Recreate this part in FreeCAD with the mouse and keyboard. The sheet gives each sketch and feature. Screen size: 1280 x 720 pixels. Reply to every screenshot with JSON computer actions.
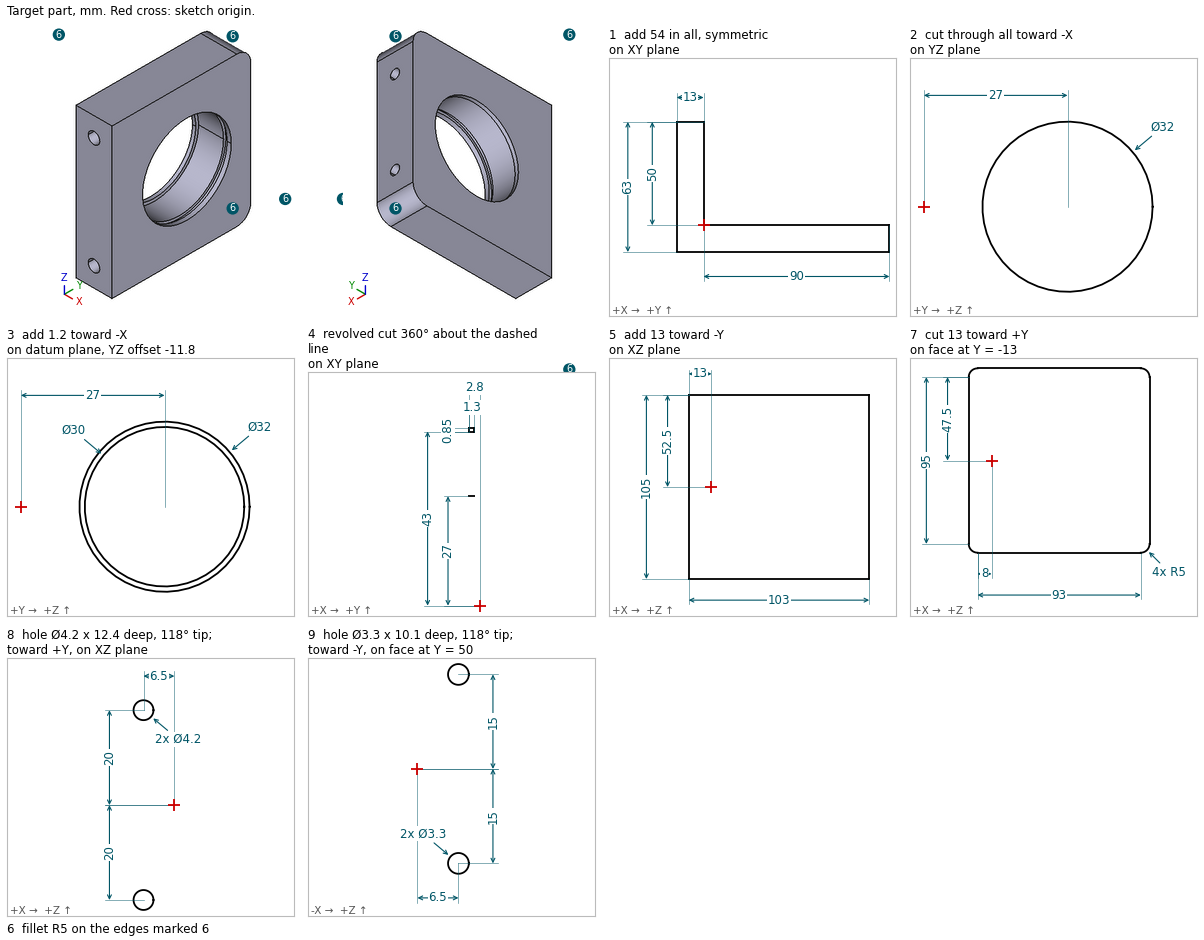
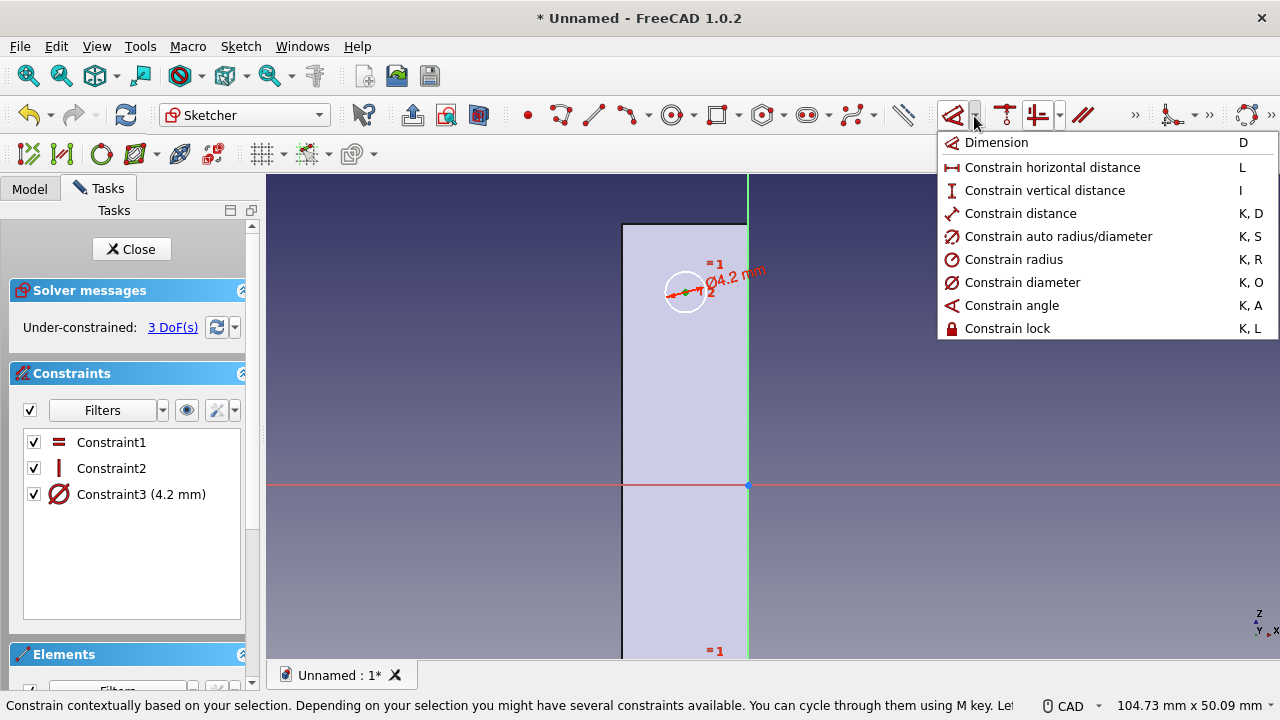
{"action": "left_click", "coordinate": [1108, 190]}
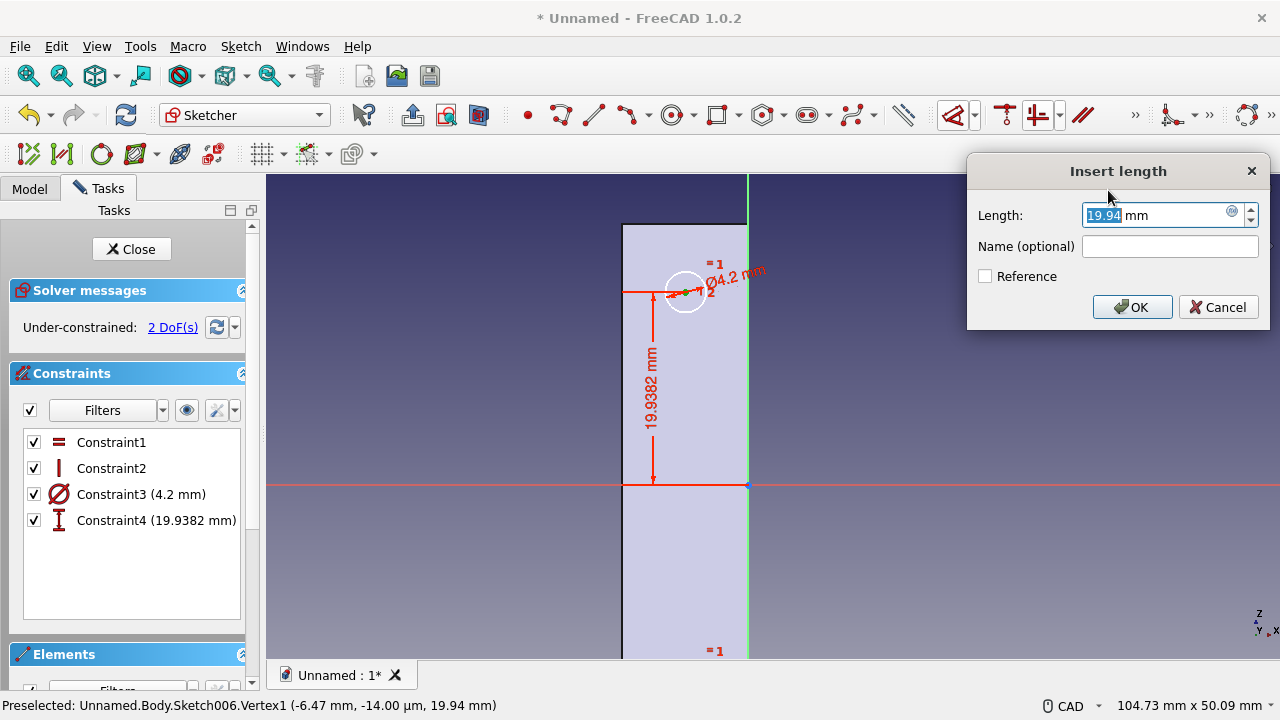
{"action": "type", "text": "20"}
{"action": "key", "text": "Return"}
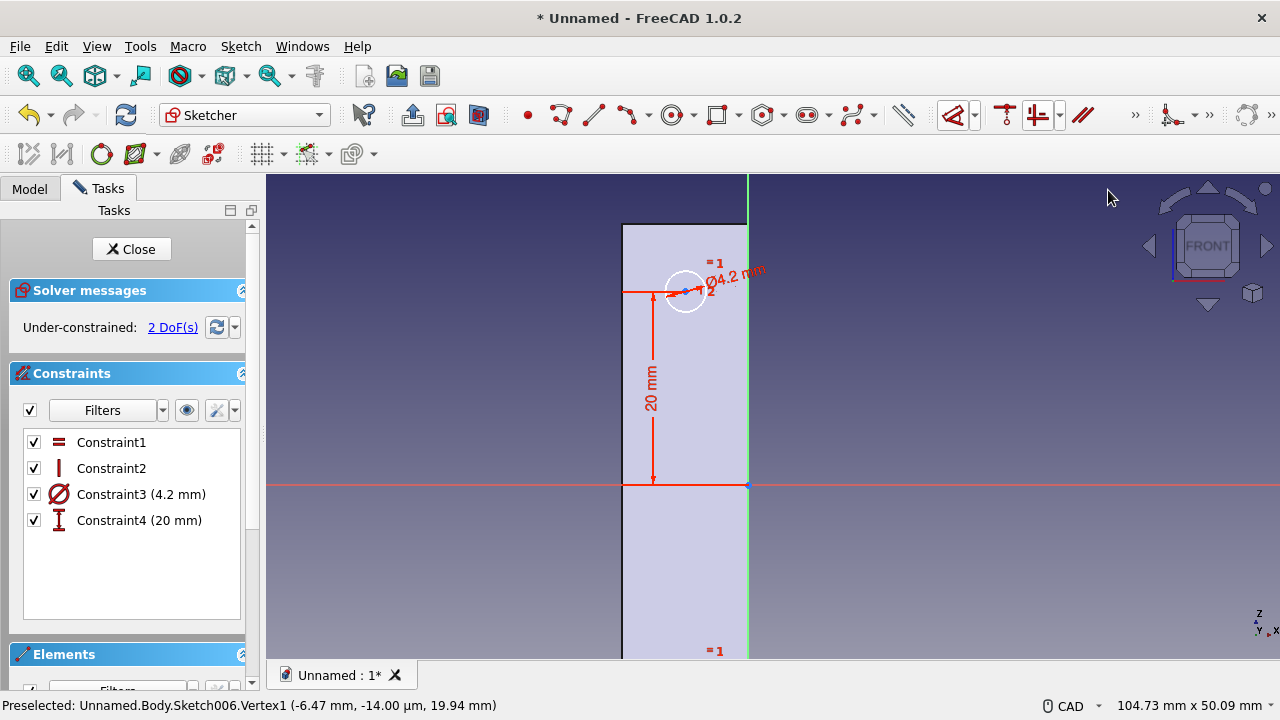
{"action": "scroll", "coordinate": [700, 277], "scroll_direction": "down", "scroll_amount": 2}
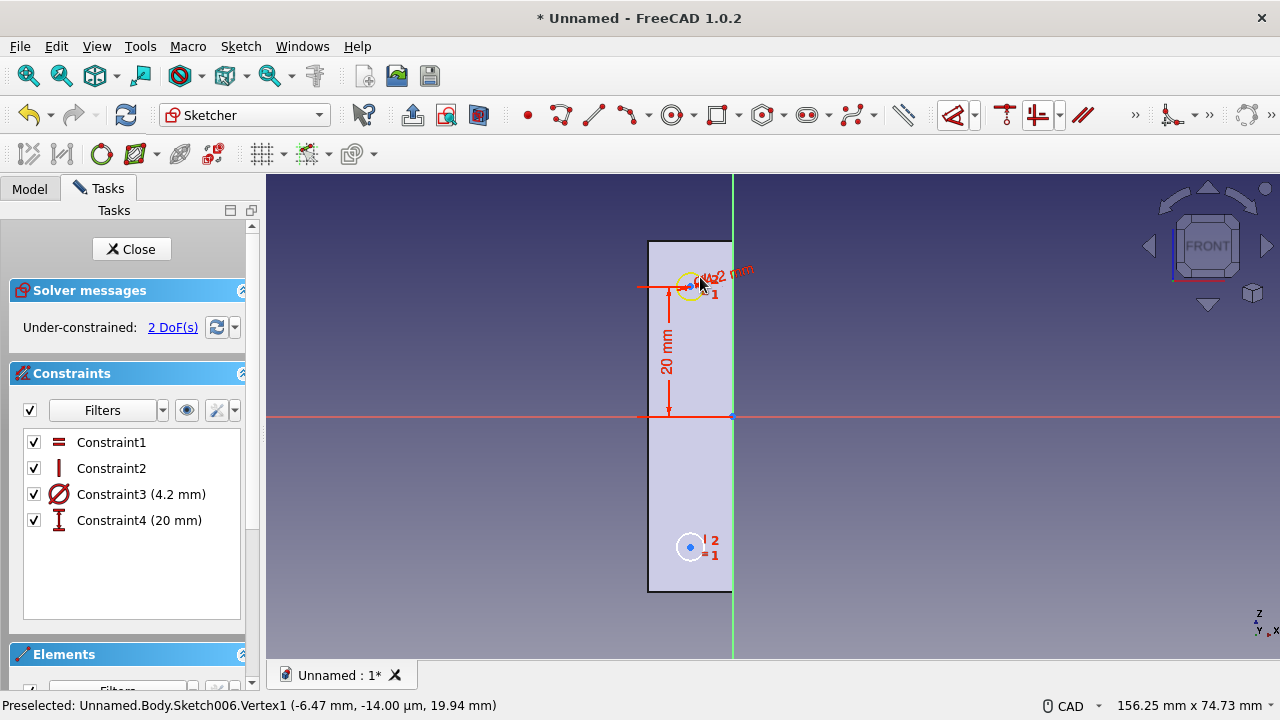
{"action": "left_click", "coordinate": [691, 547]}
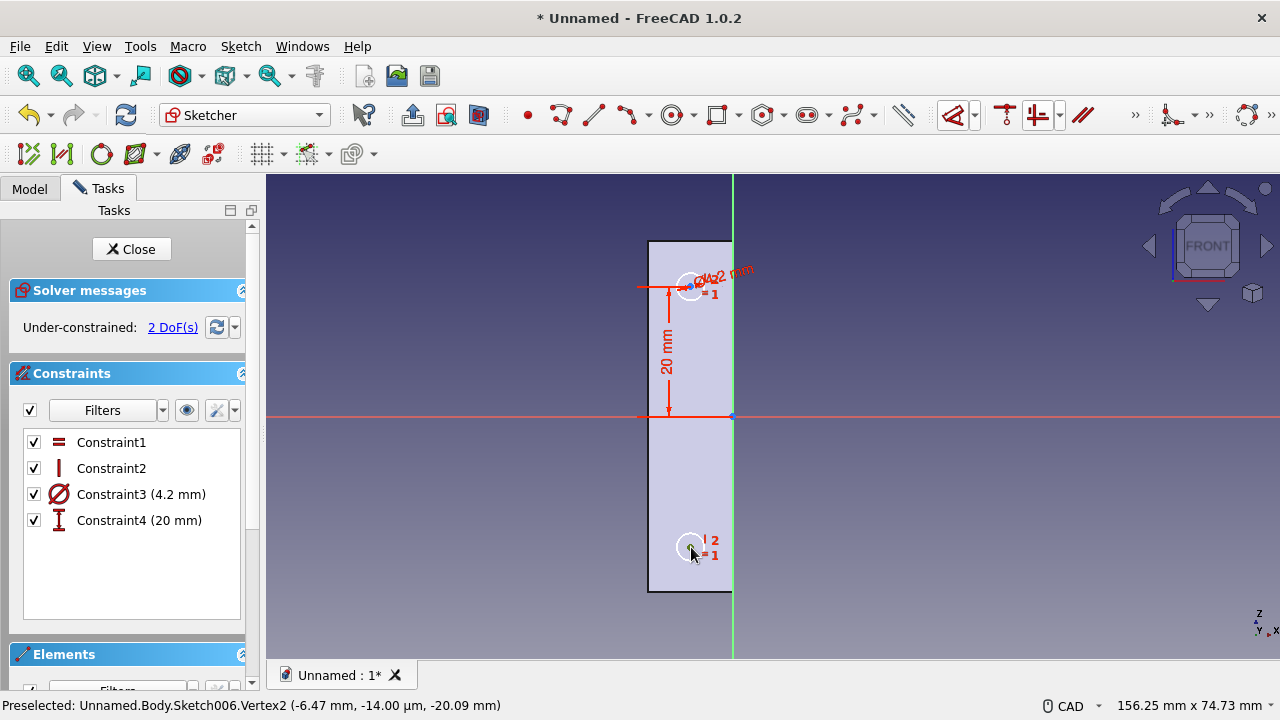
{"action": "left_click", "coordinate": [974, 116]}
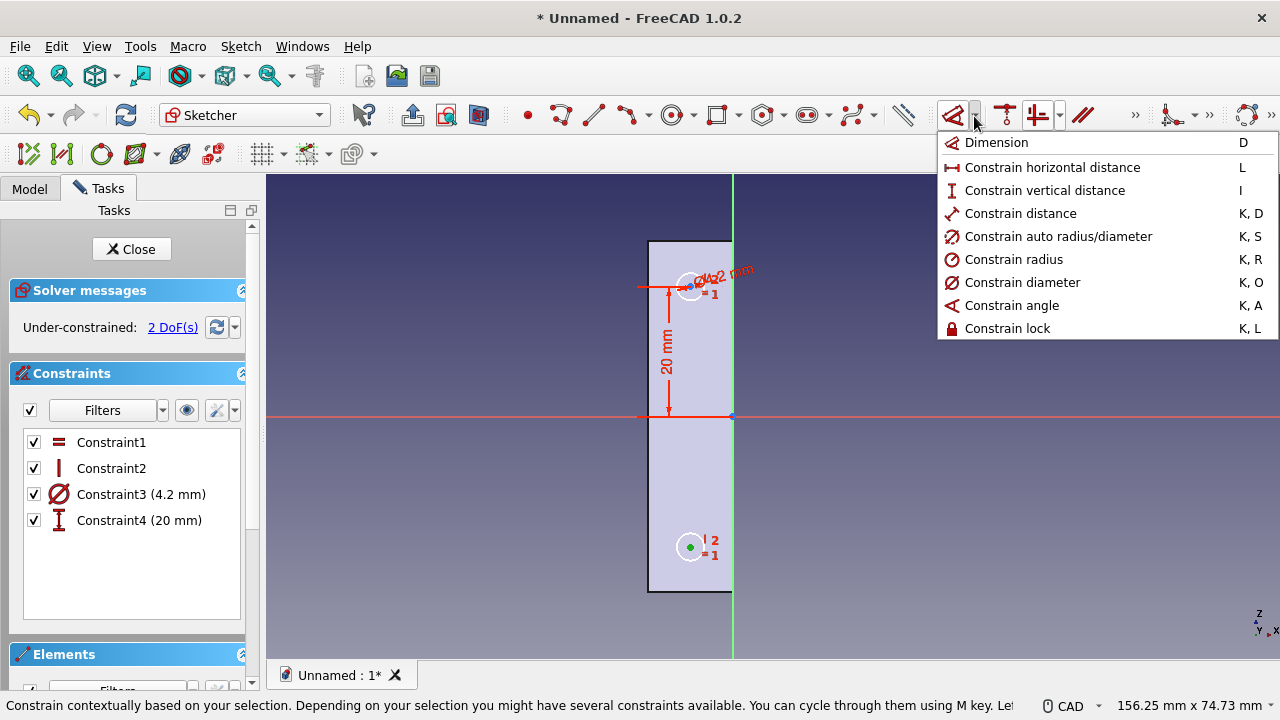
{"action": "left_click", "coordinate": [1108, 190]}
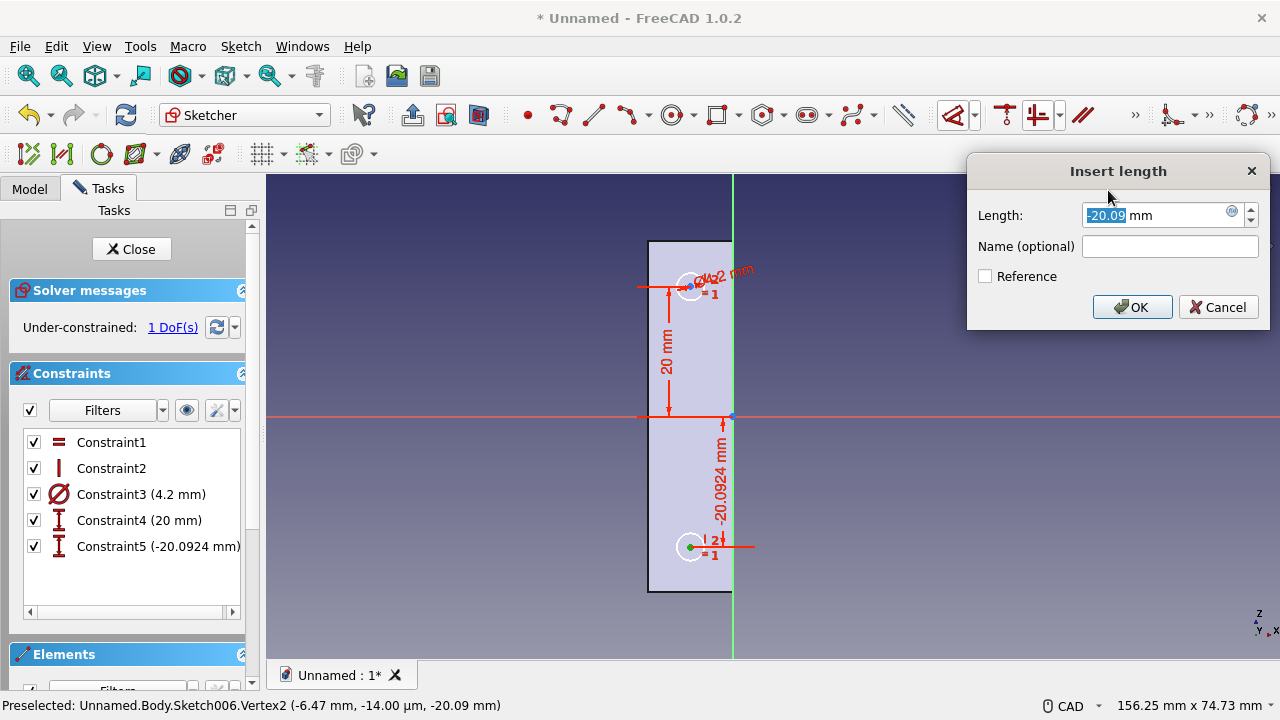
{"action": "type", "text": "-20"}
{"action": "key", "text": "Return"}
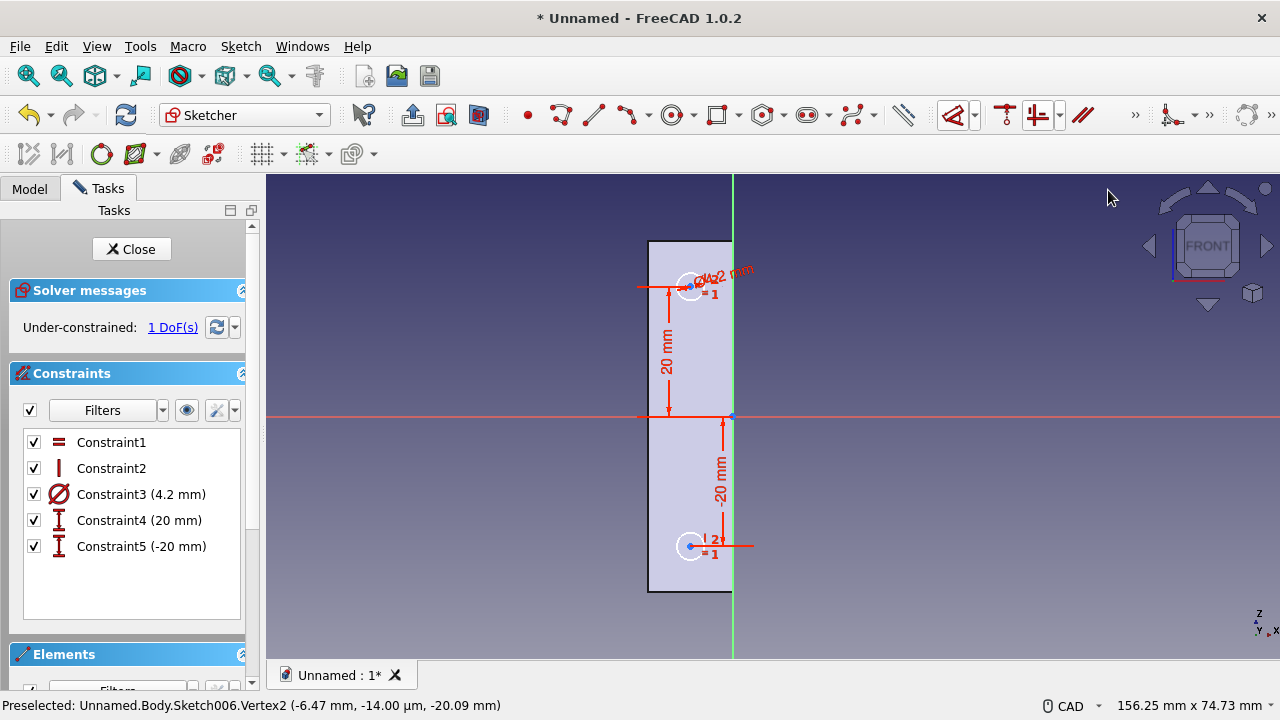
{"action": "left_click", "coordinate": [691, 287]}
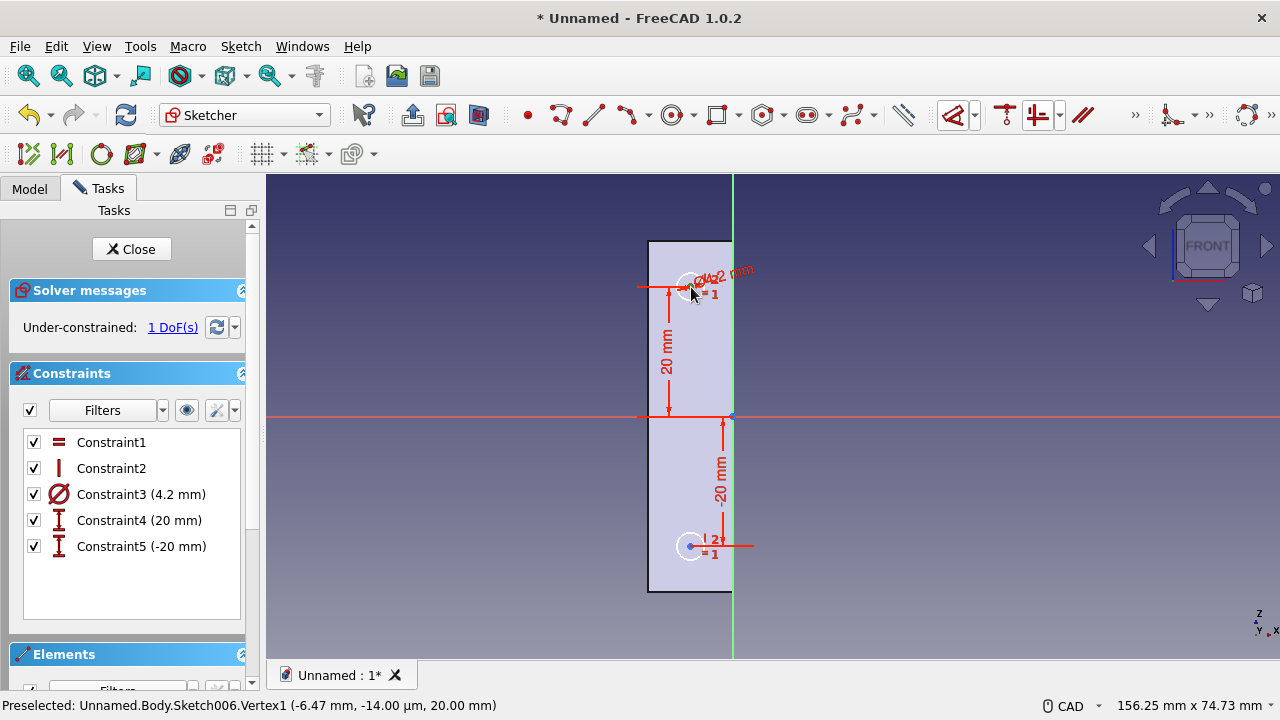
{"action": "left_click", "coordinate": [974, 116]}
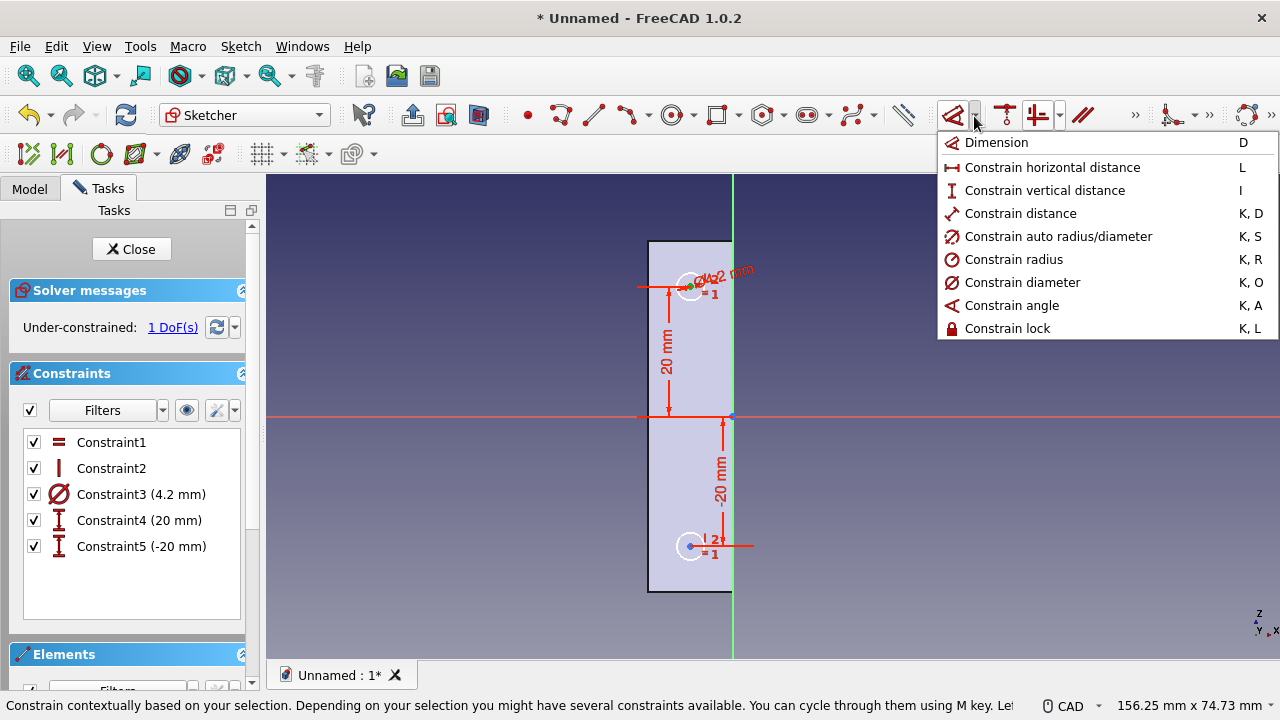
{"action": "left_click", "coordinate": [1108, 168]}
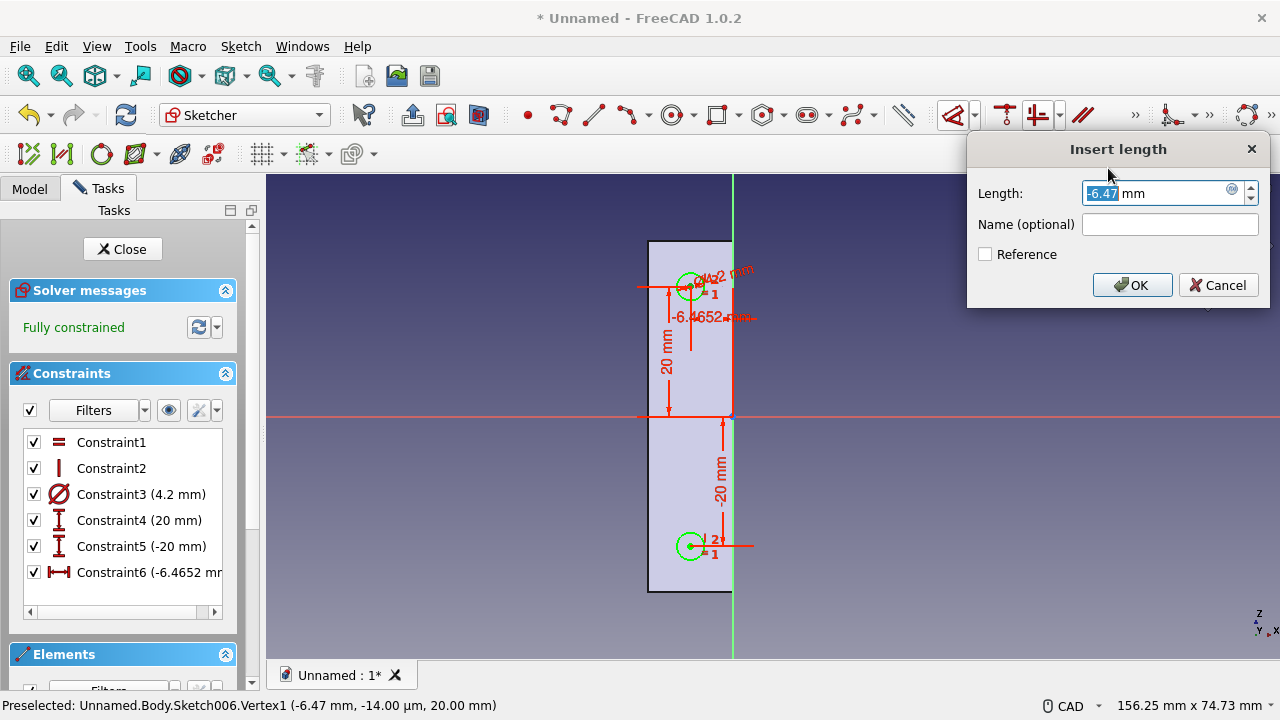
{"action": "type", "text": "-6.5"}
{"action": "key", "text": "Return"}